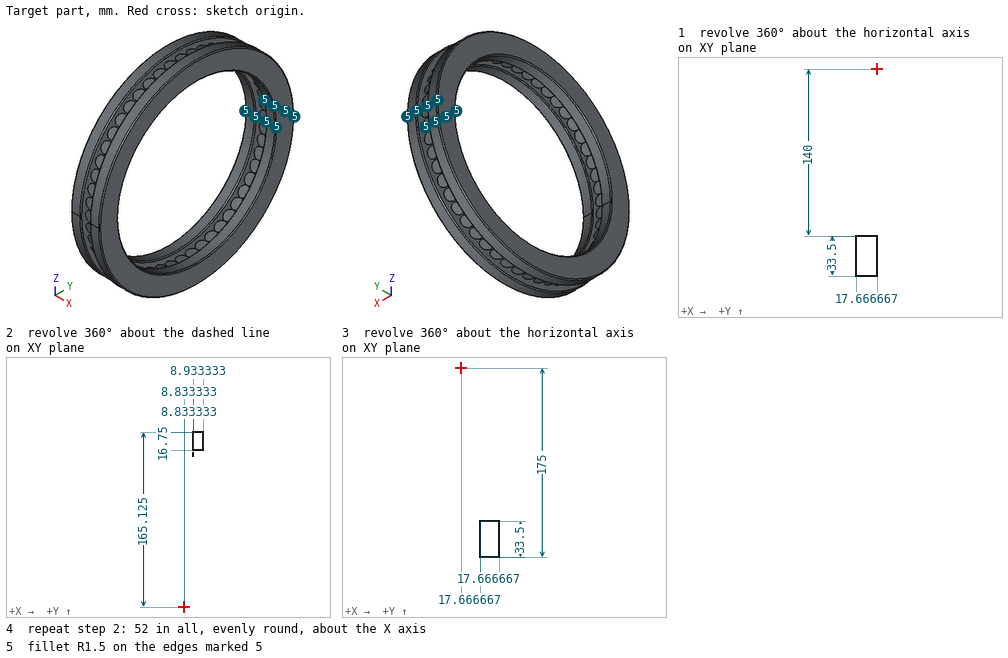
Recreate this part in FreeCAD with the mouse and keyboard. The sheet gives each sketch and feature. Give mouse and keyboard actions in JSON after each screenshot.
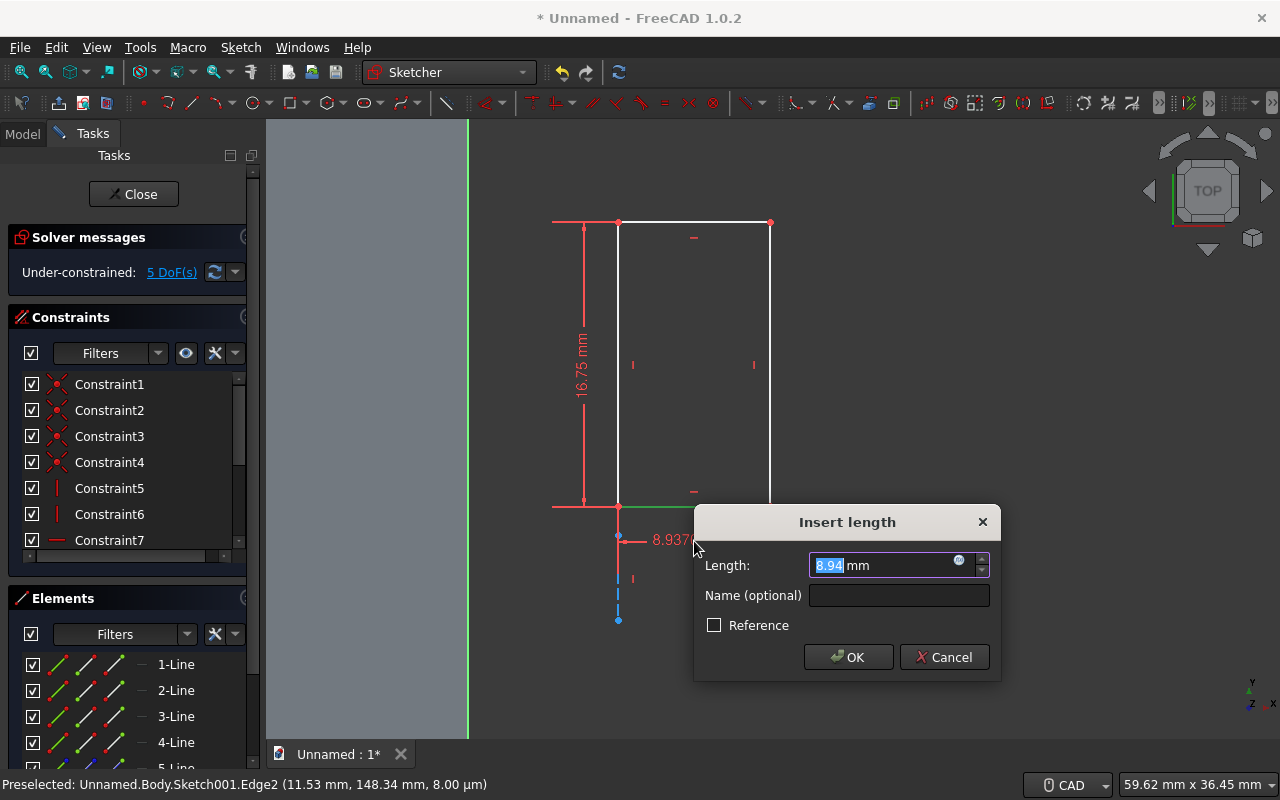
{"action": "type", "text": "8.933333"}
{"action": "key", "text": "Return"}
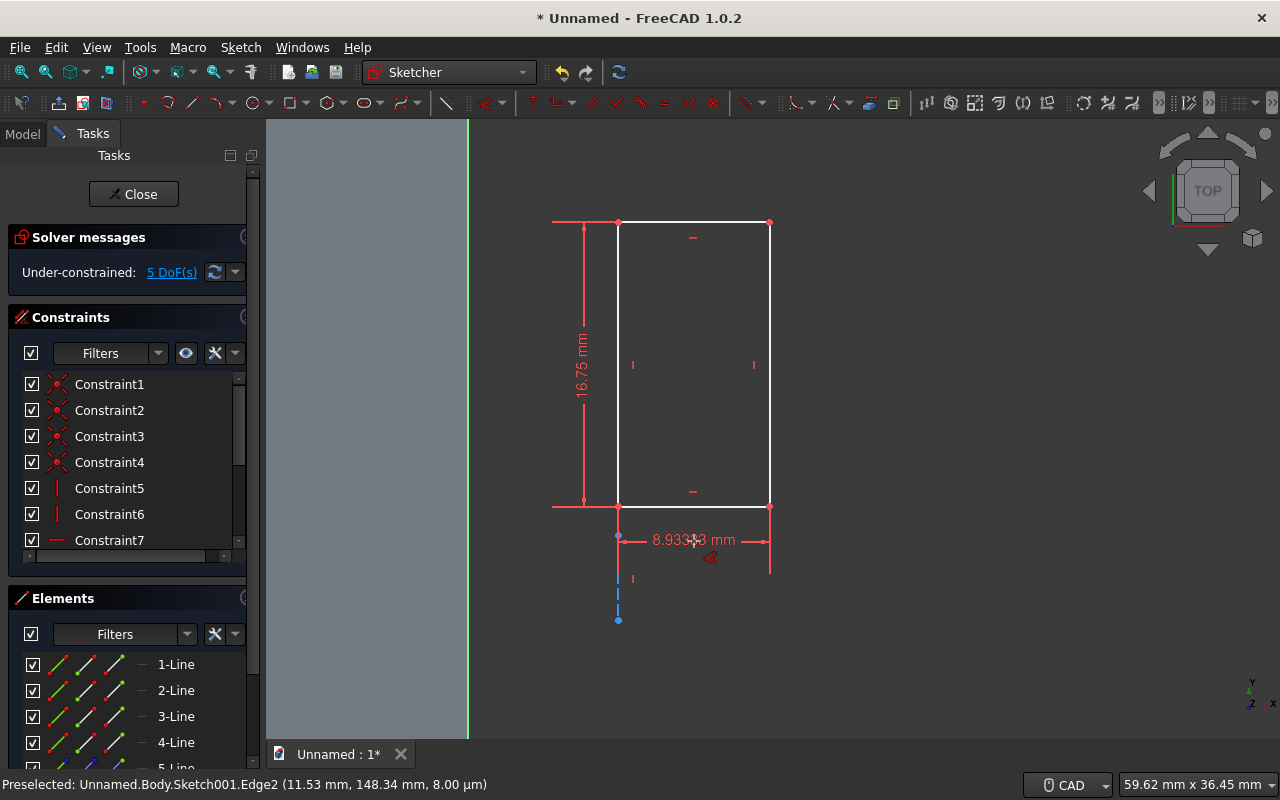
{"action": "left_click", "coordinate": [618, 222]}
{"action": "left_click", "coordinate": [434, 467]}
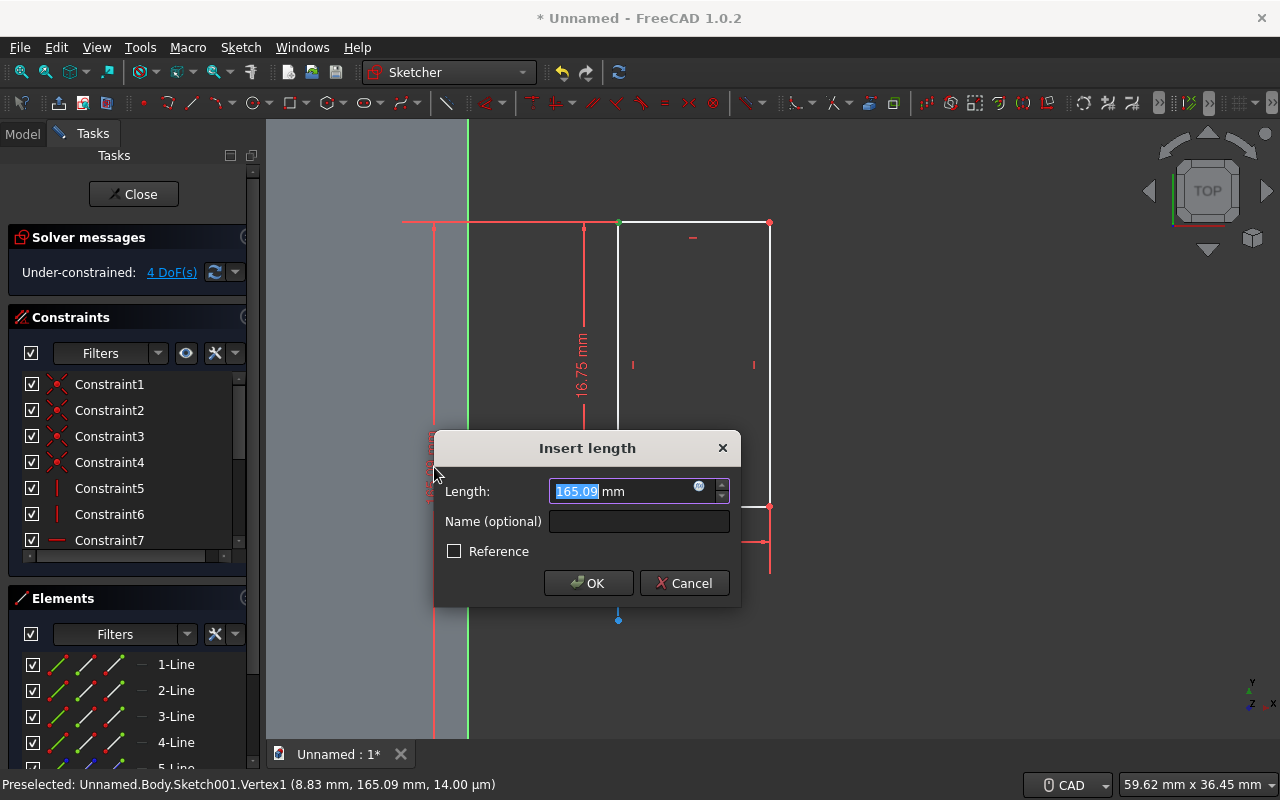
{"action": "type", "text": "165.125"}
{"action": "key", "text": "Return"}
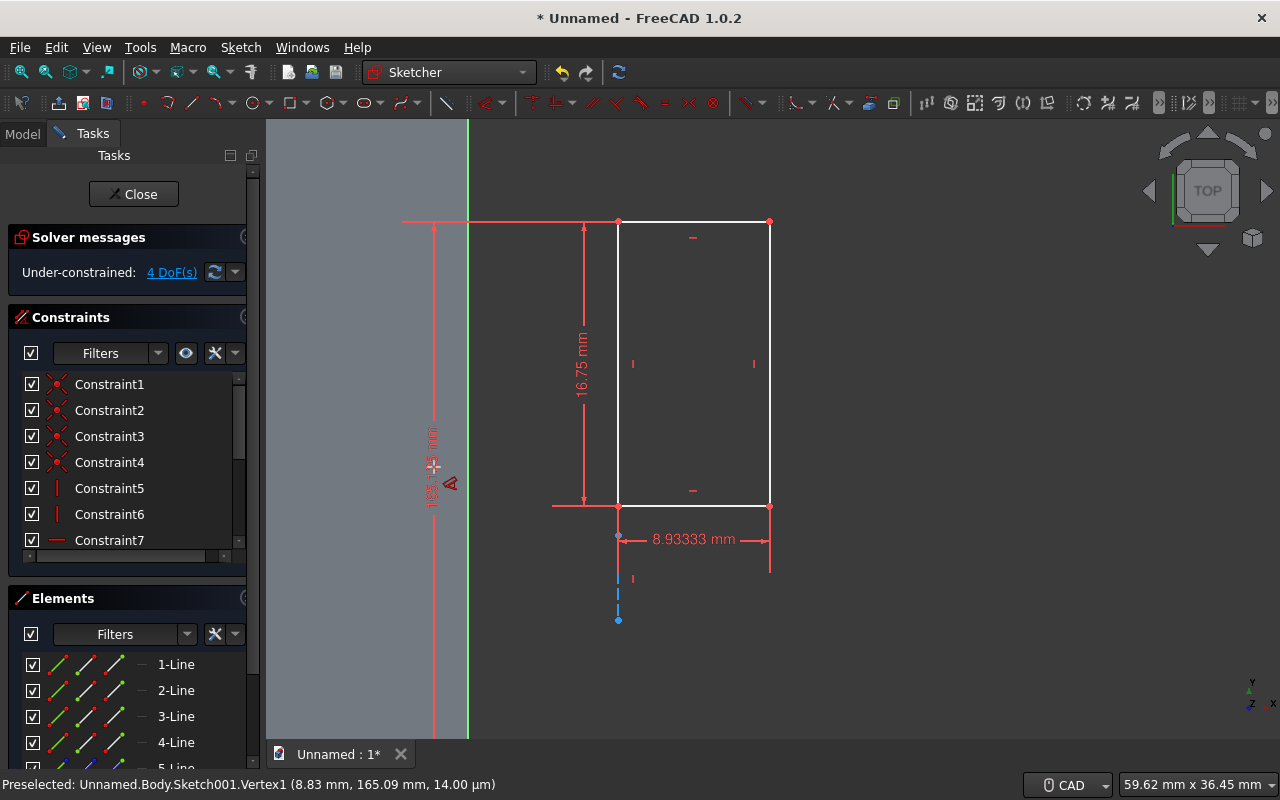
{"action": "left_click", "coordinate": [618, 222]}
{"action": "left_click", "coordinate": [543, 188]}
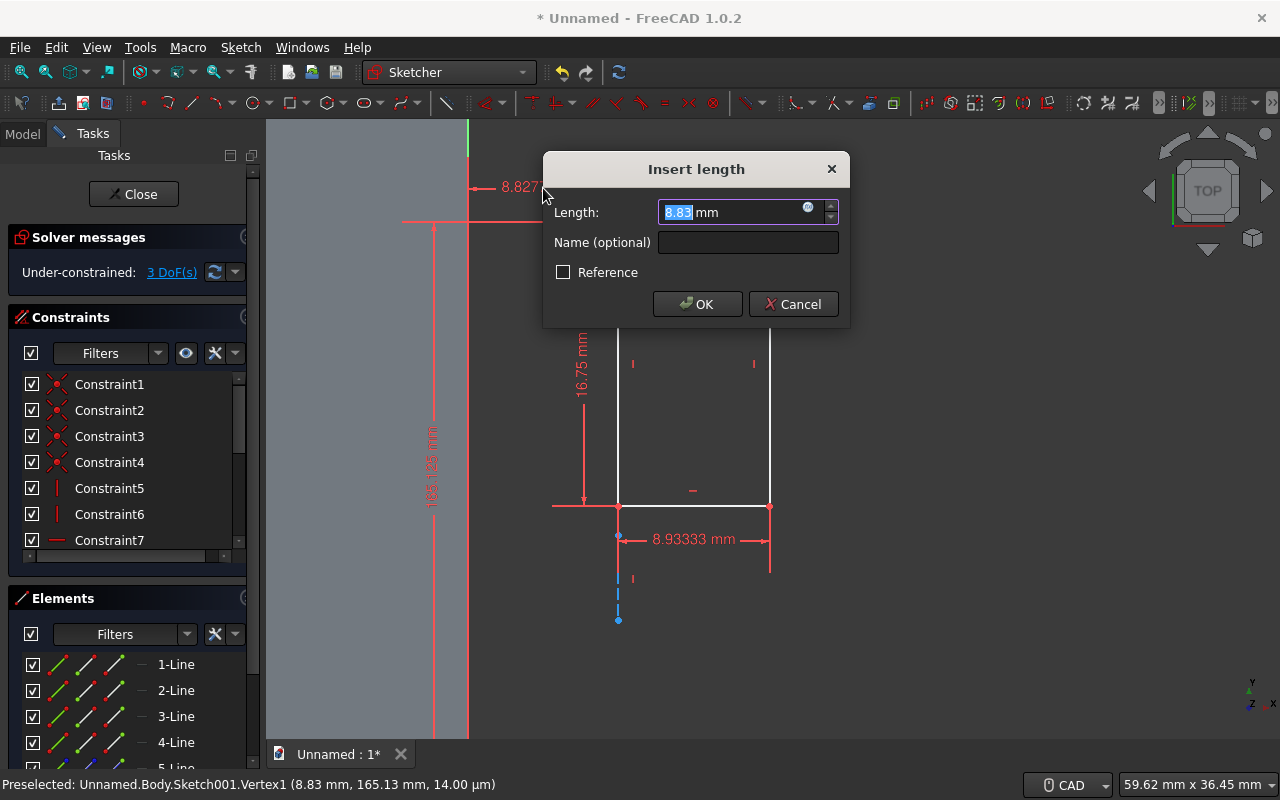
{"action": "type", "text": "8.833333"}
{"action": "key", "text": "Return"}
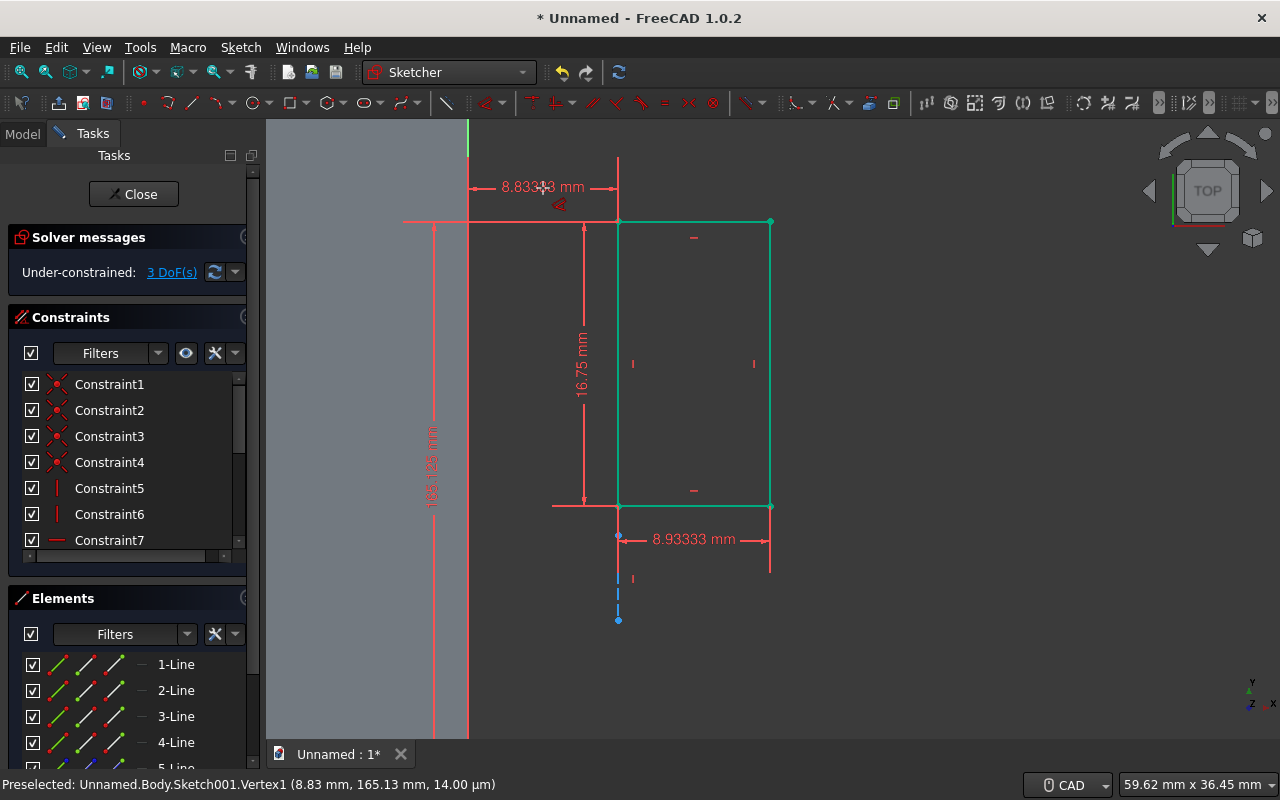
{"action": "left_click", "coordinate": [618, 536]}
{"action": "left_click", "coordinate": [543, 502]}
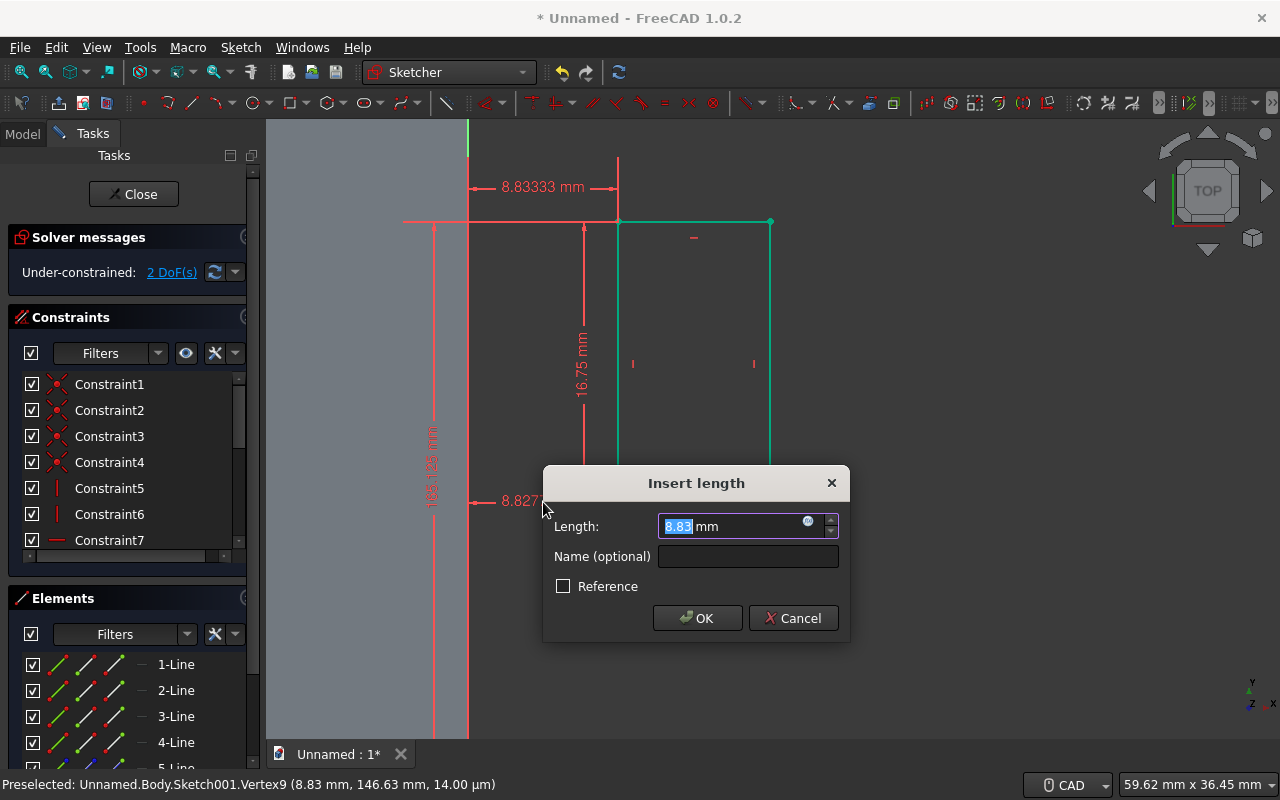
{"action": "type", "text": "8.833333"}
{"action": "key", "text": "Return"}
{"action": "key", "text": "Escape"}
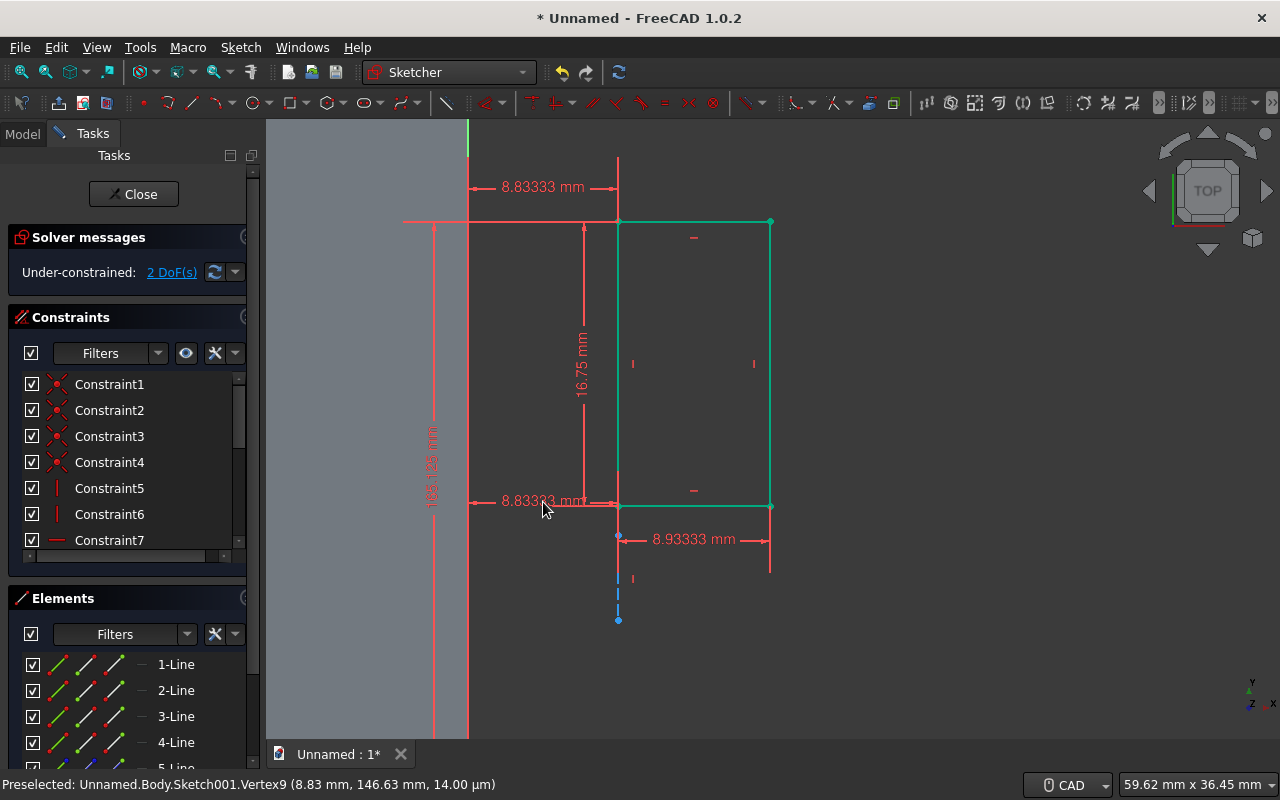
{"action": "left_click", "coordinate": [134, 194]}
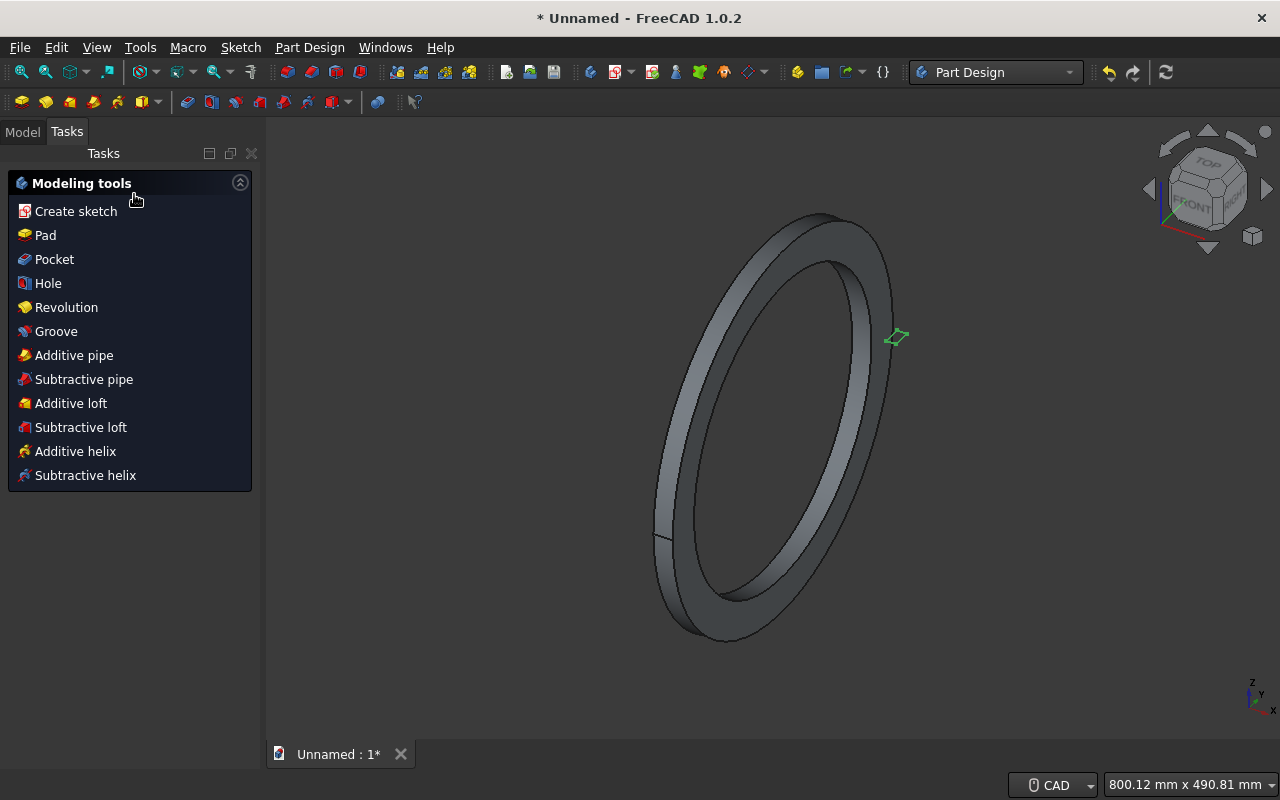
{"action": "left_click", "coordinate": [46, 102]}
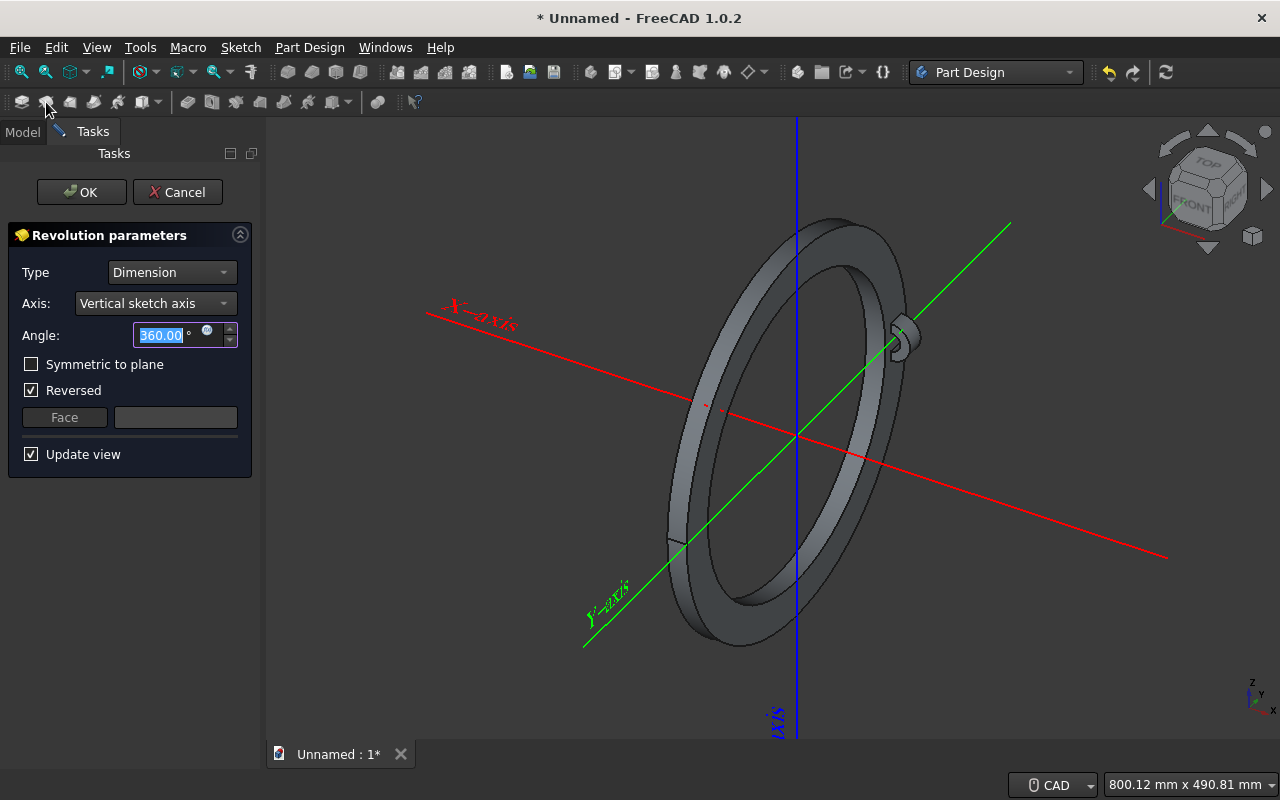
{"action": "left_click", "coordinate": [156, 304]}